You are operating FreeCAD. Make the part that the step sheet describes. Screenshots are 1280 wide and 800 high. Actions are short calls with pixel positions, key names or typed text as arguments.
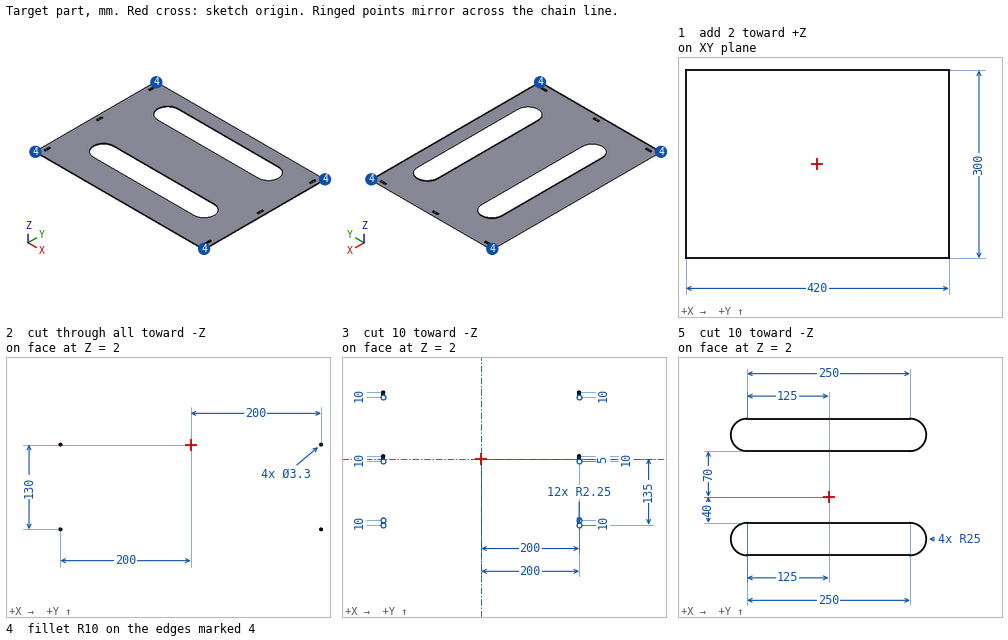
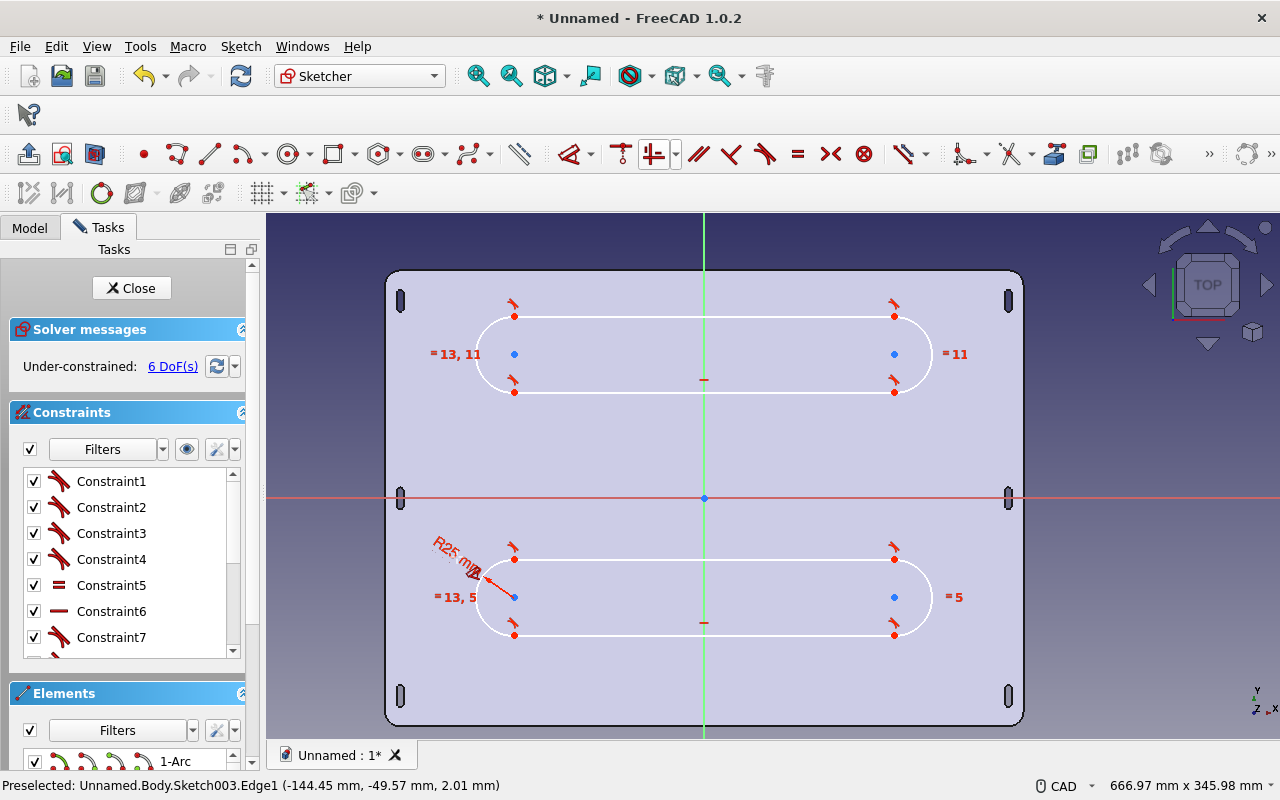
click(628, 560)
click(617, 594)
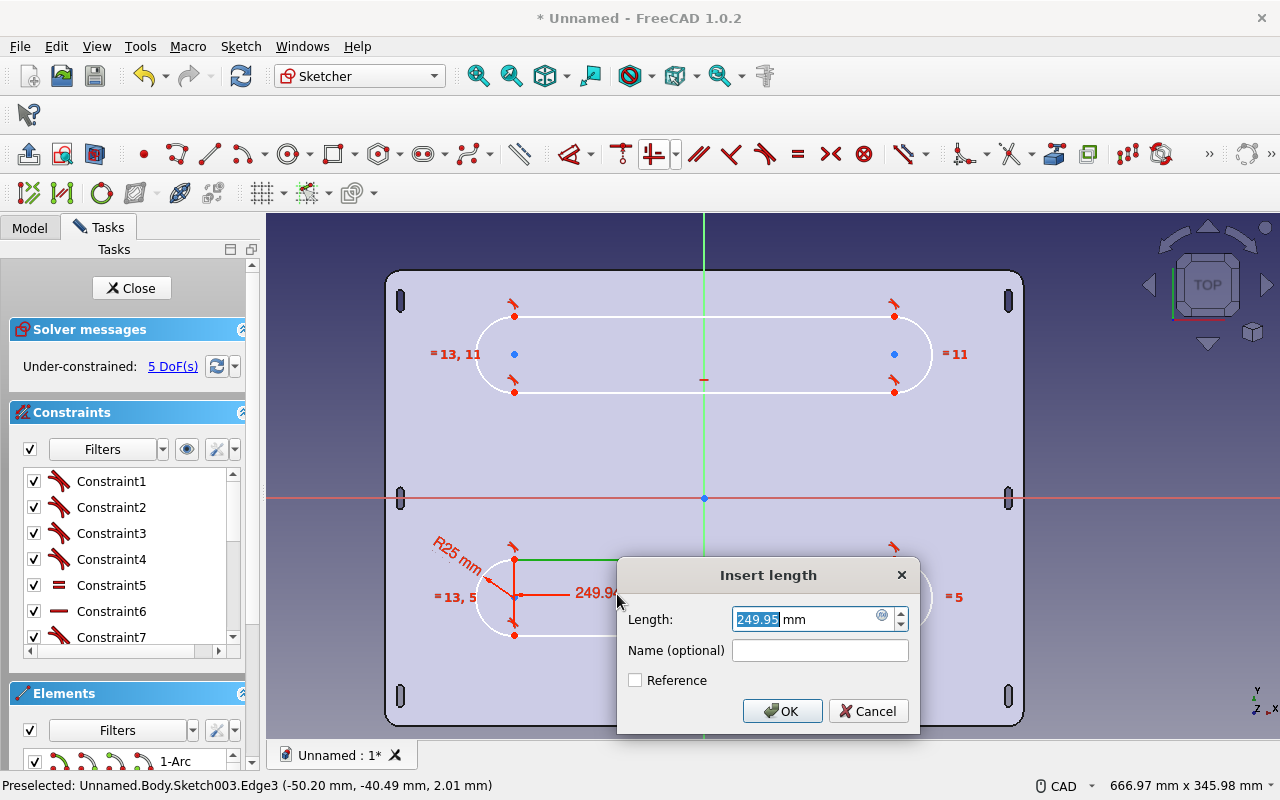
text(250)
key(Return)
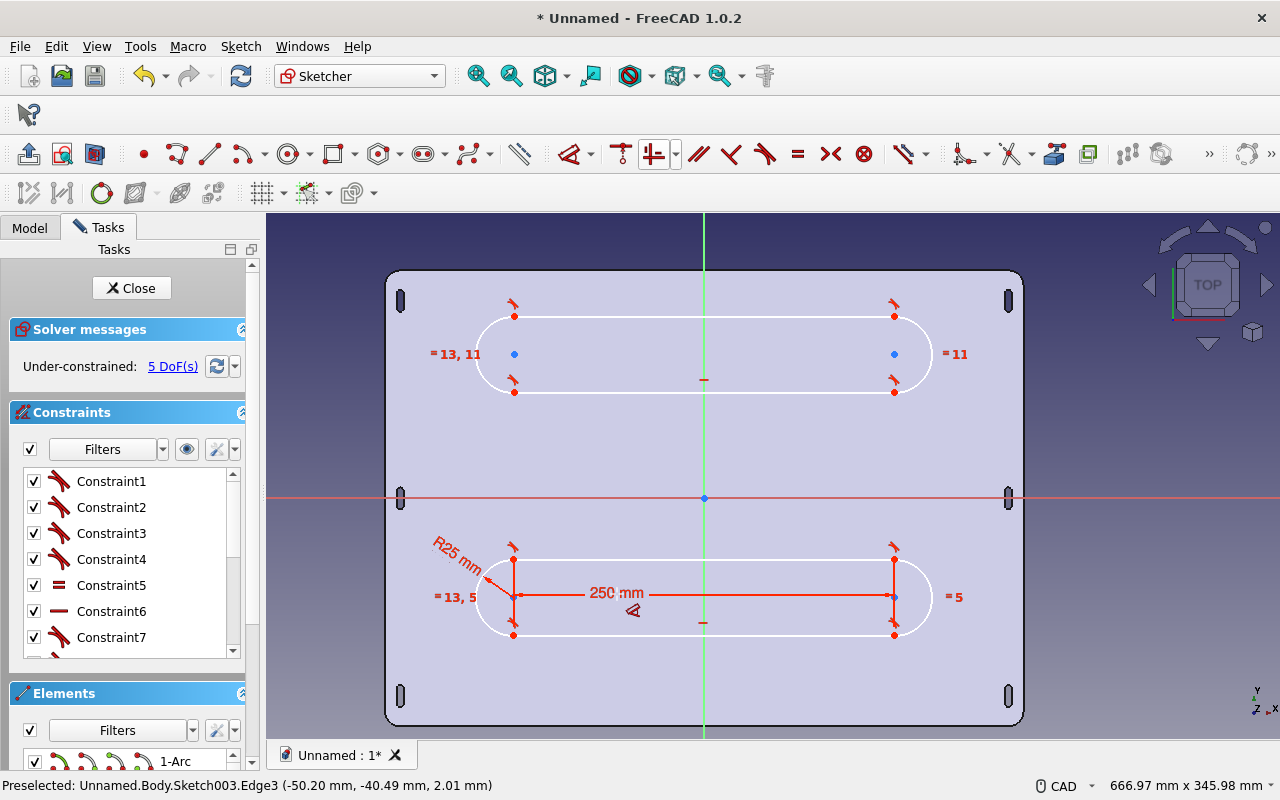
click(628, 317)
click(617, 283)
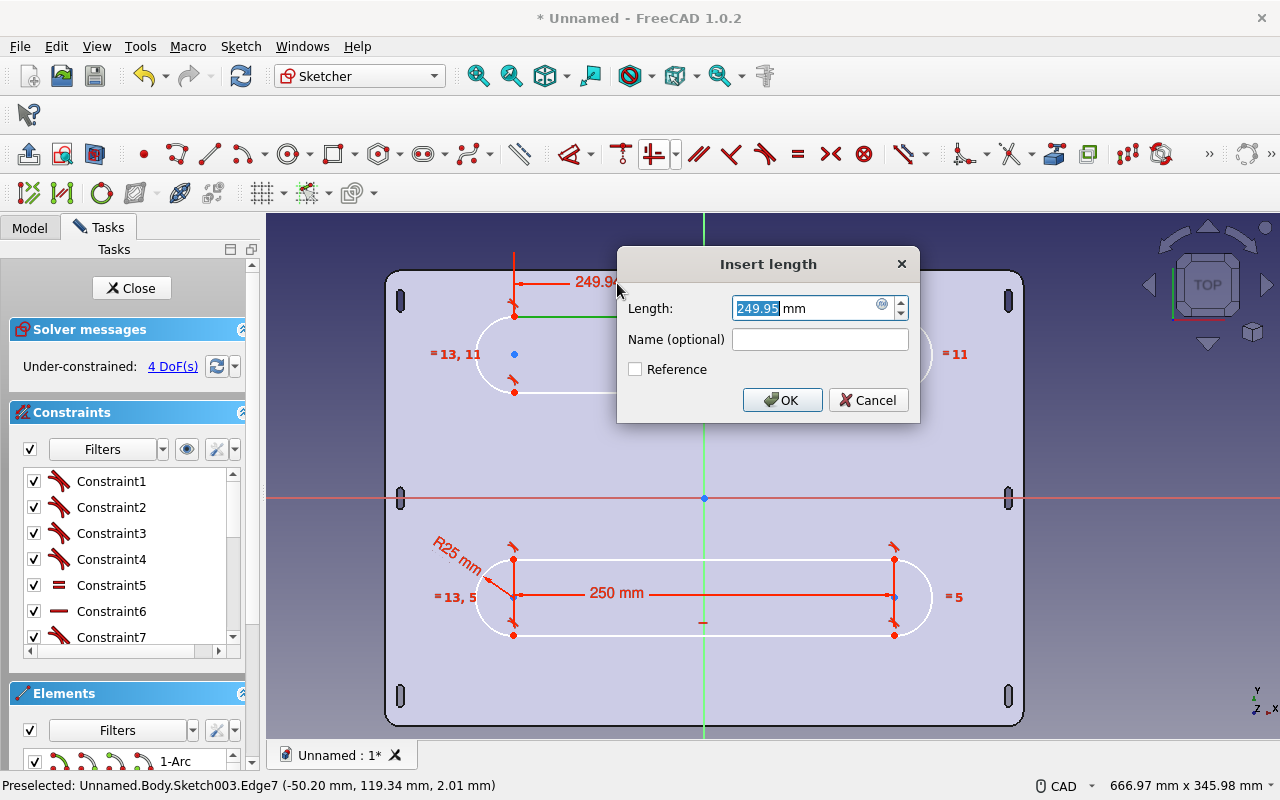
text(250)
key(Return)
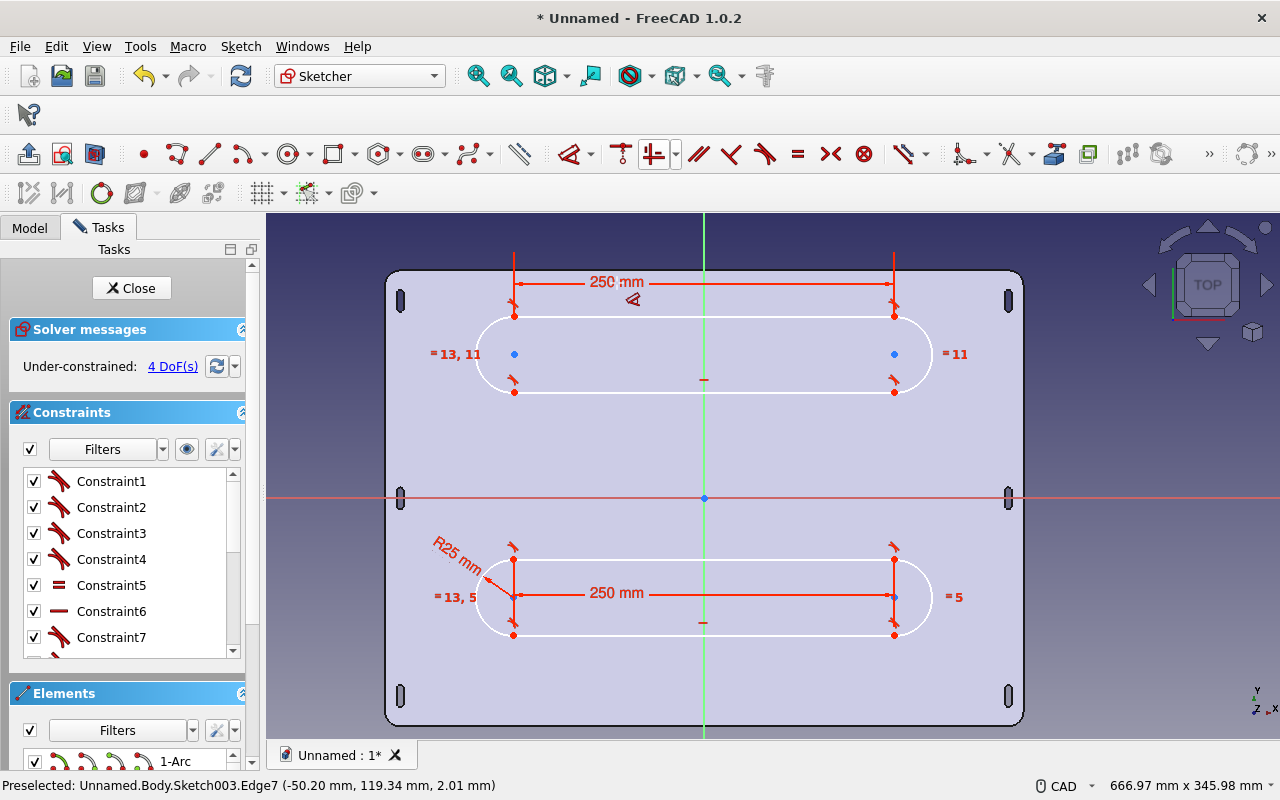
click(514, 560)
click(480, 529)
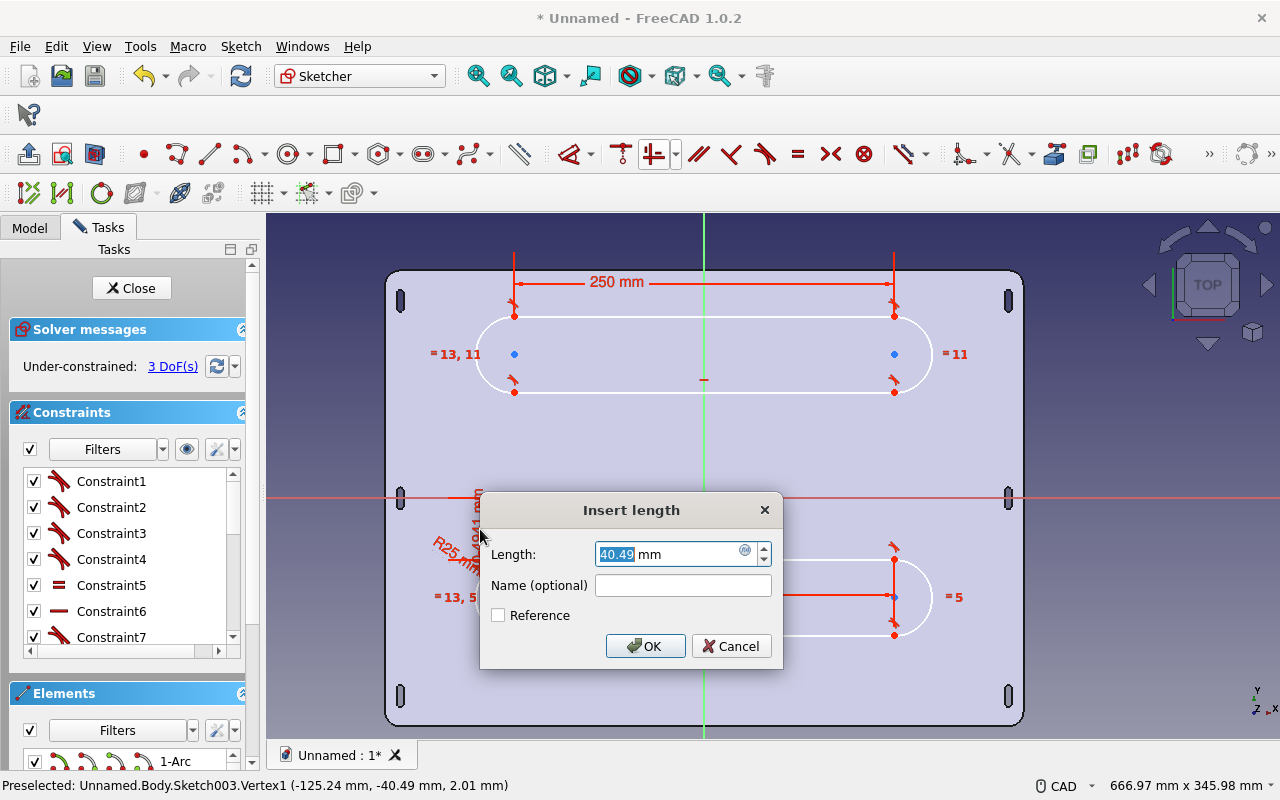
text(40)
key(Return)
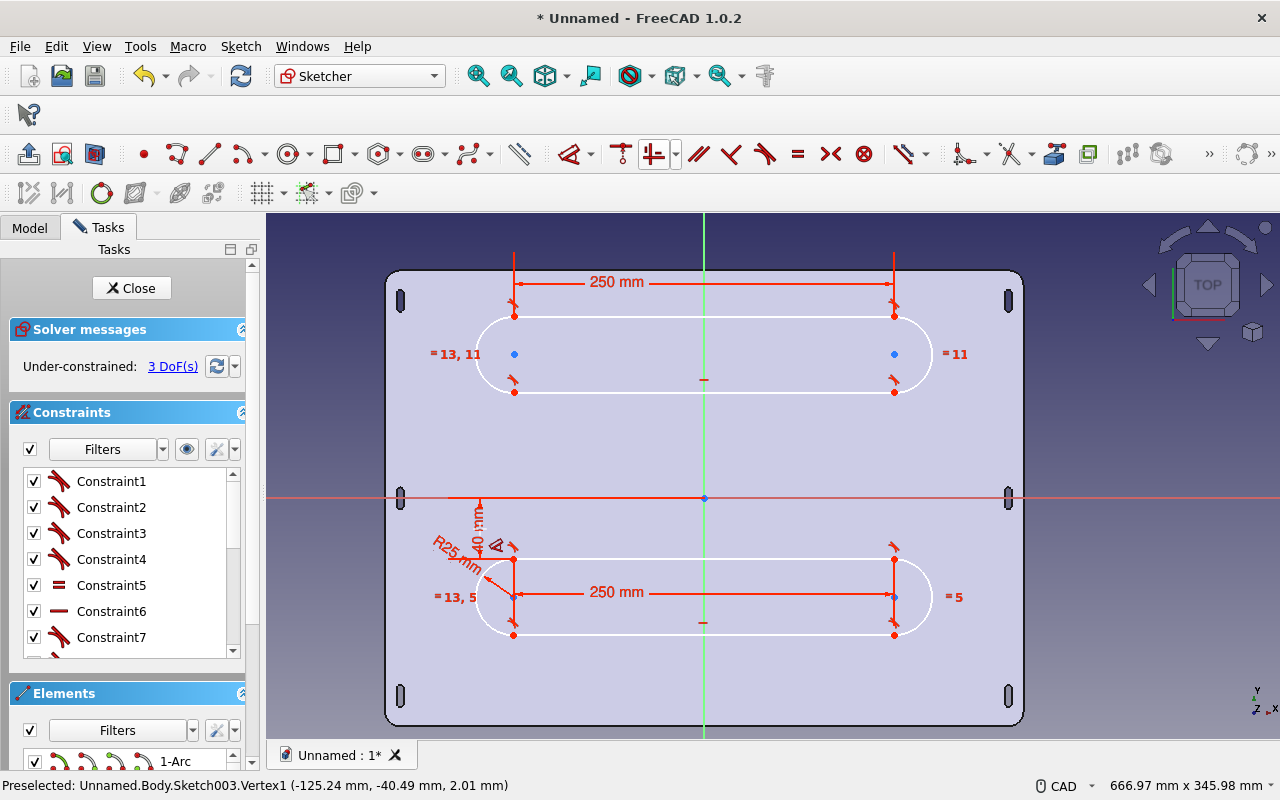
click(514, 393)
click(480, 446)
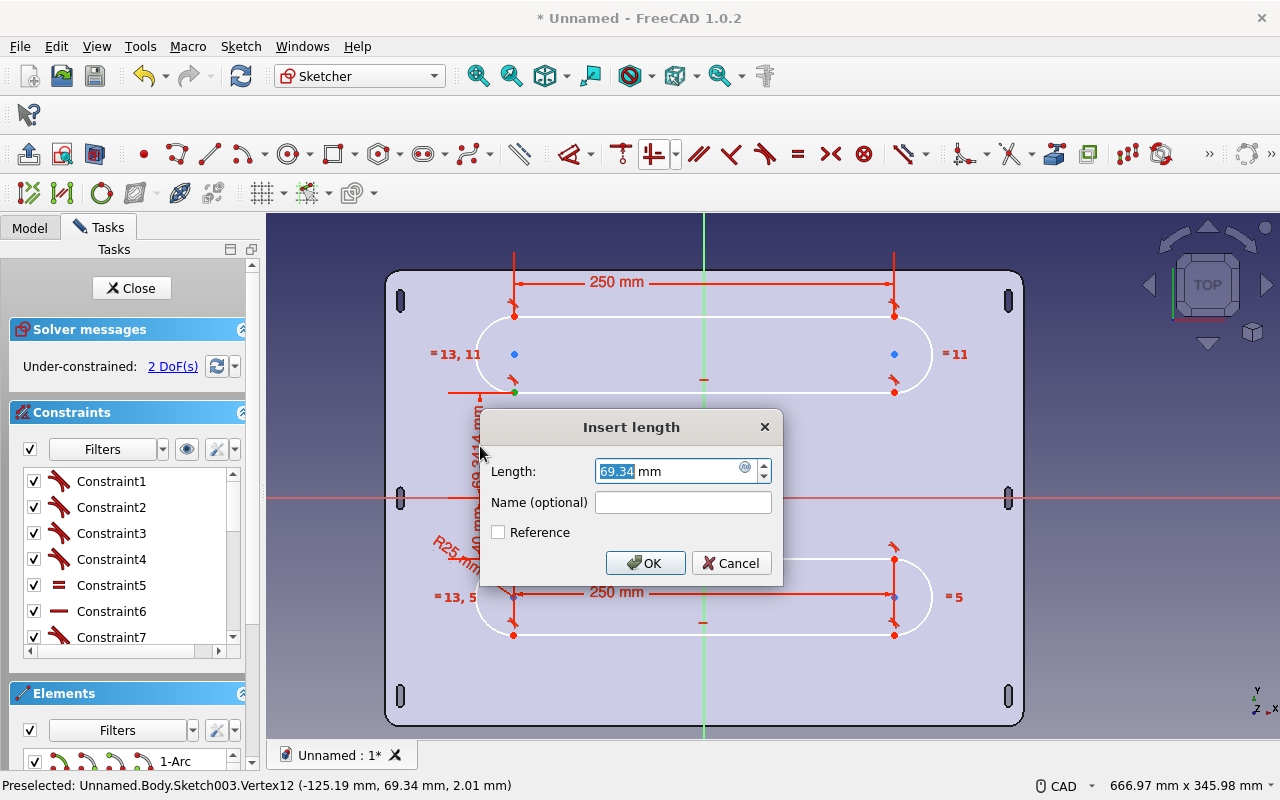
text(70)
key(Return)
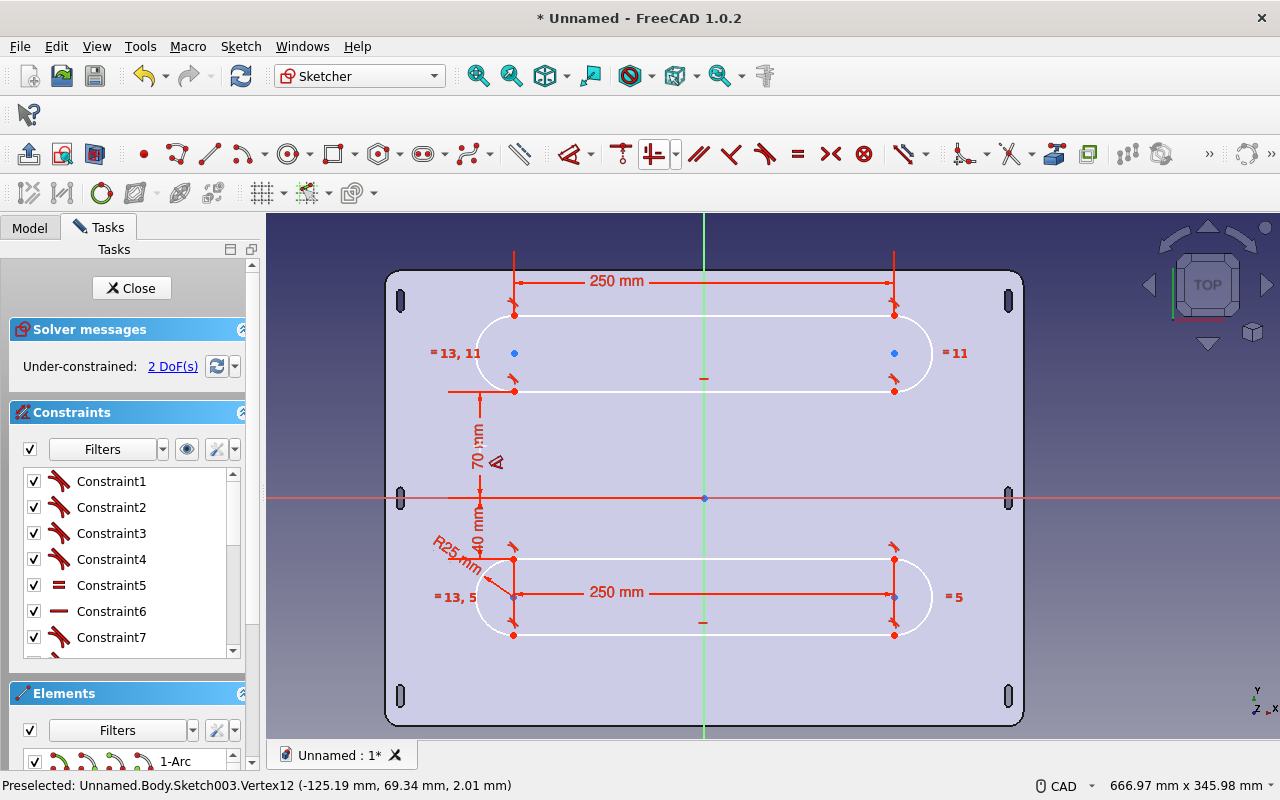
click(514, 559)
click(542, 593)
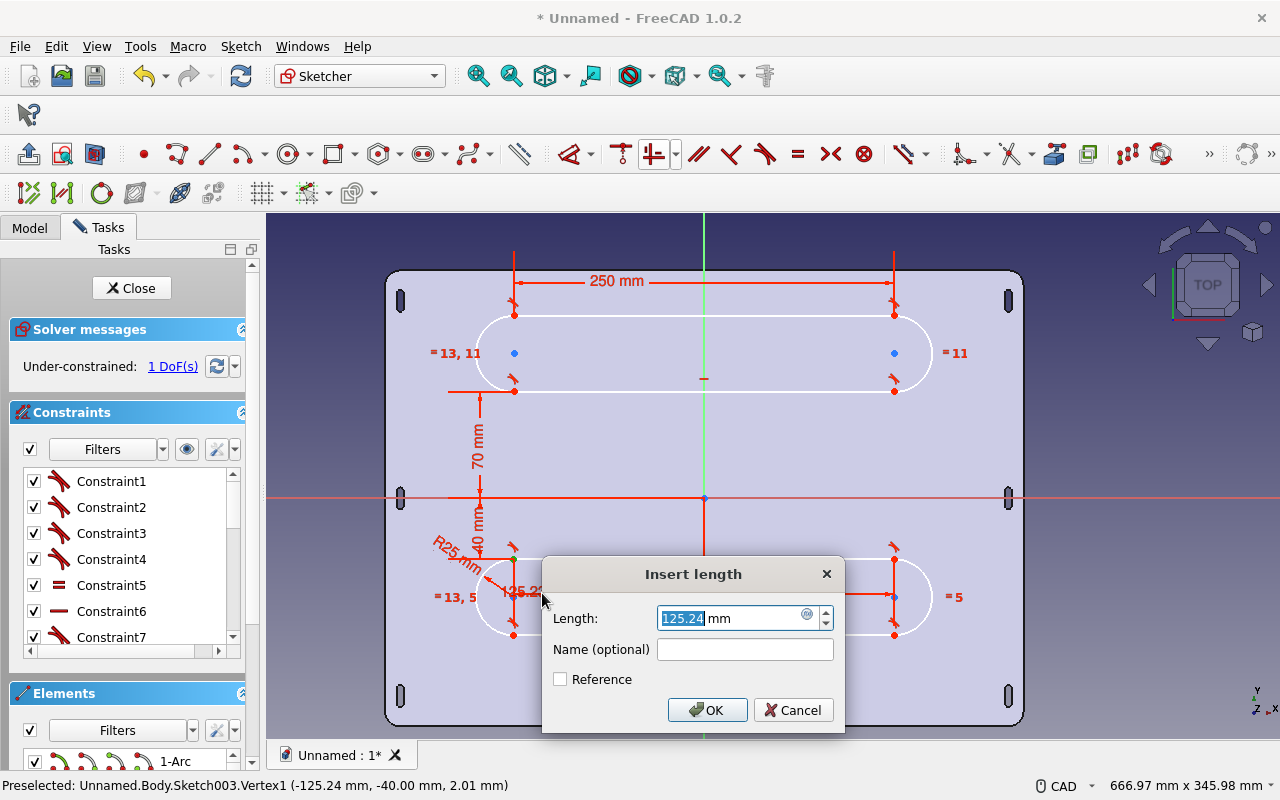
text(125)
key(Return)